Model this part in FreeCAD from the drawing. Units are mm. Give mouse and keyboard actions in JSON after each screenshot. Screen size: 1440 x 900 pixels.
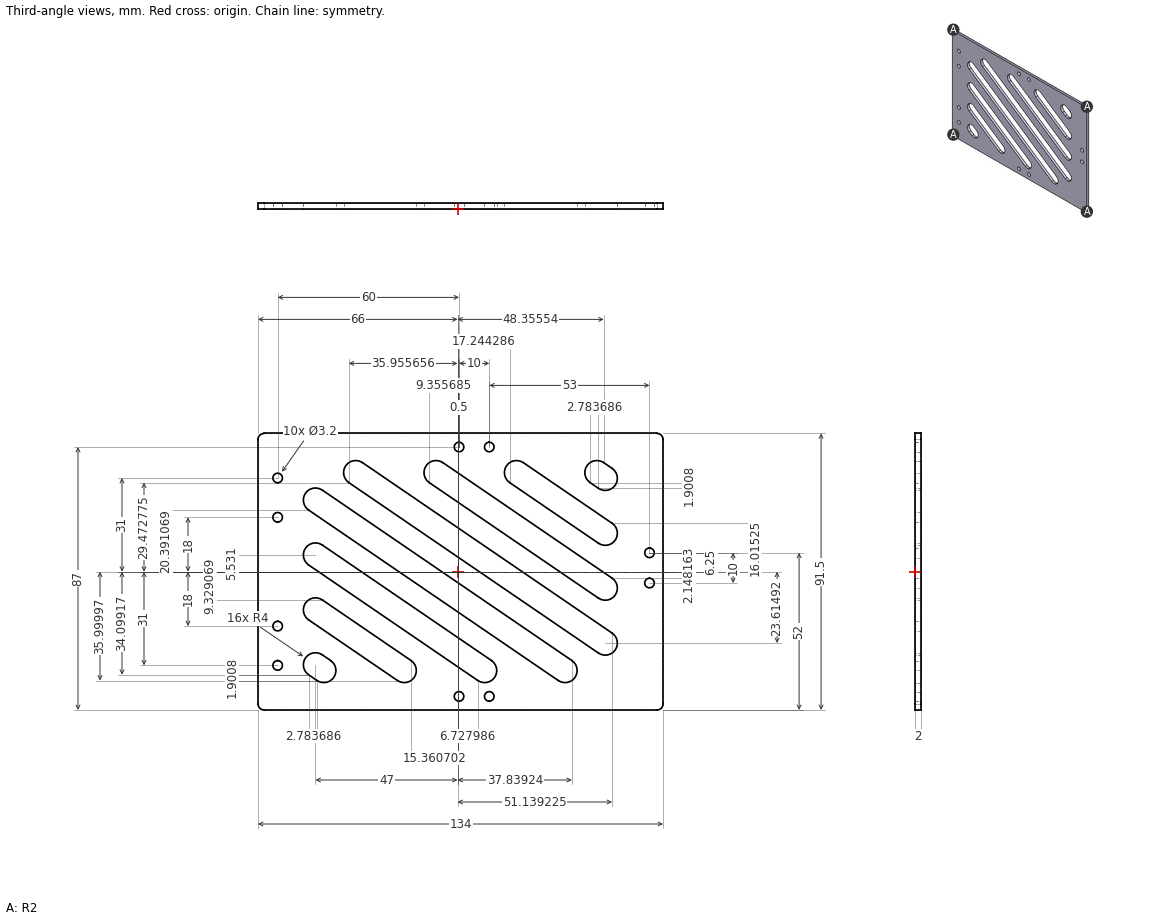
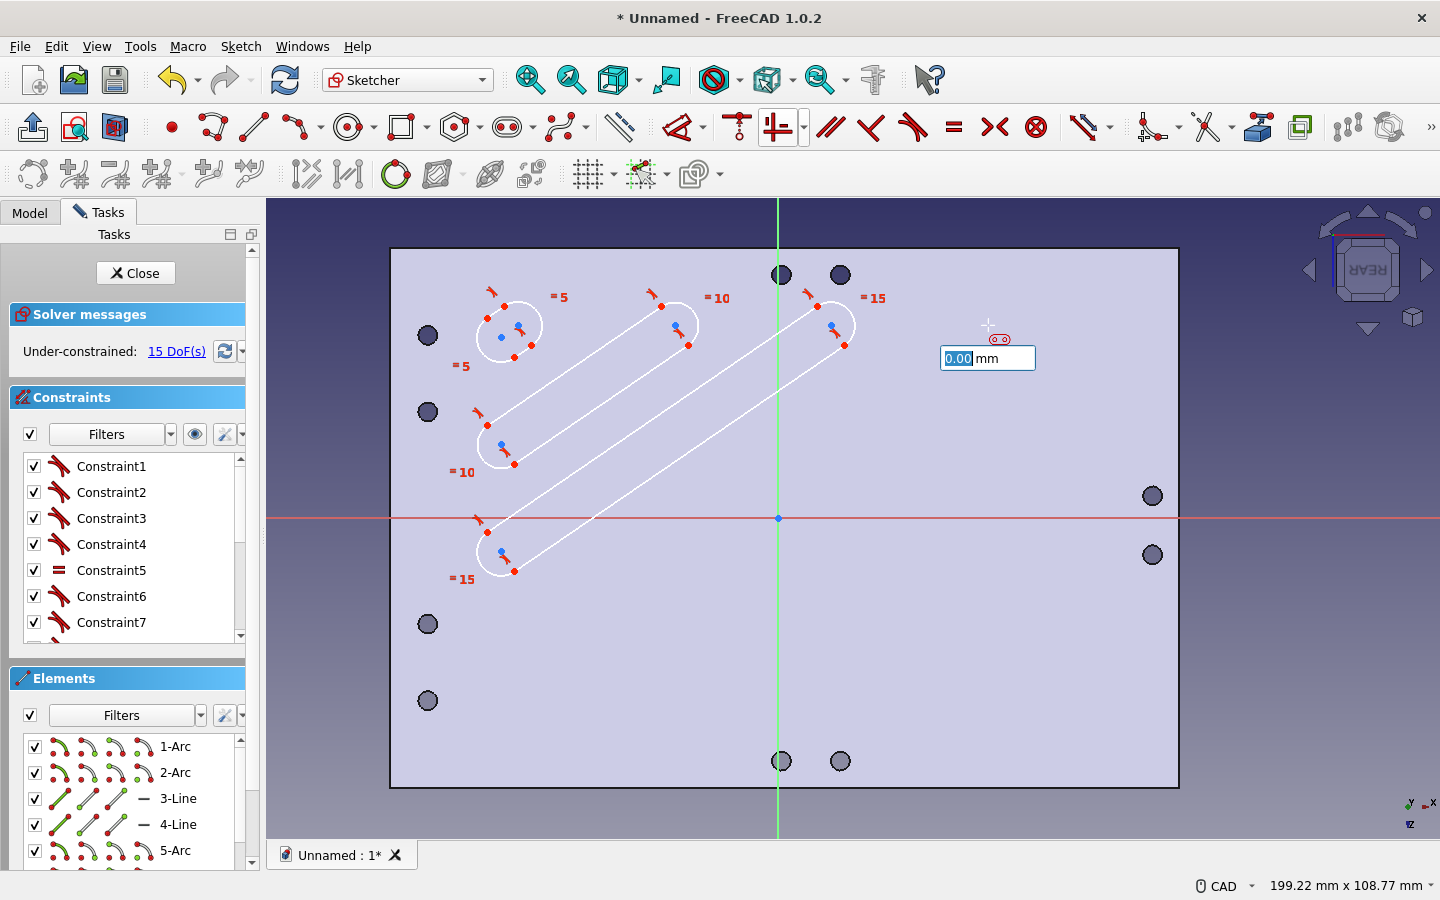
{"action": "left_click", "coordinate": [732, 472]}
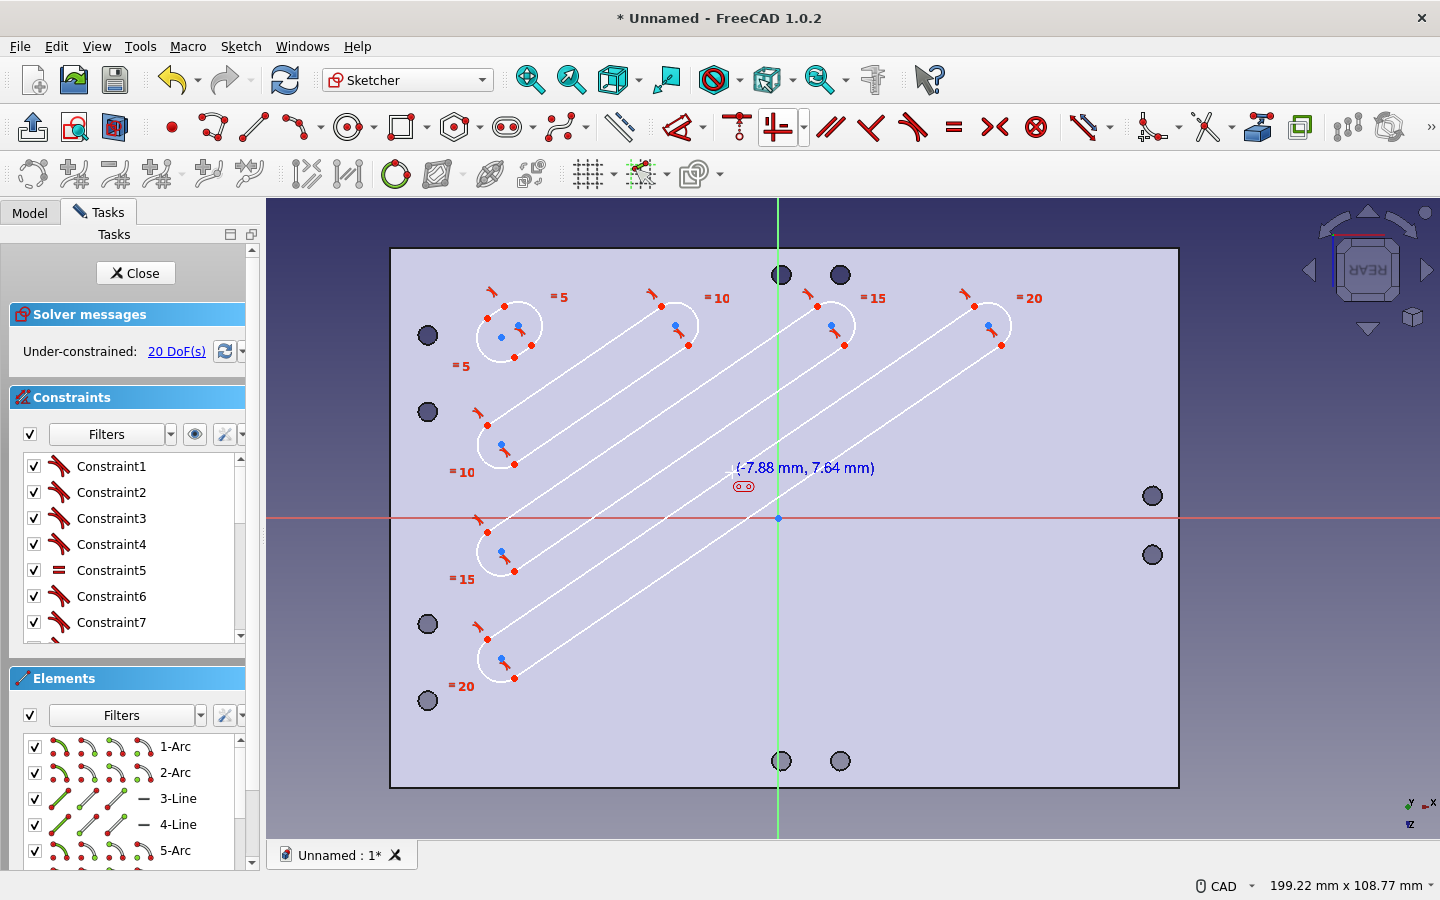
{"action": "left_click", "coordinate": [580, 711]}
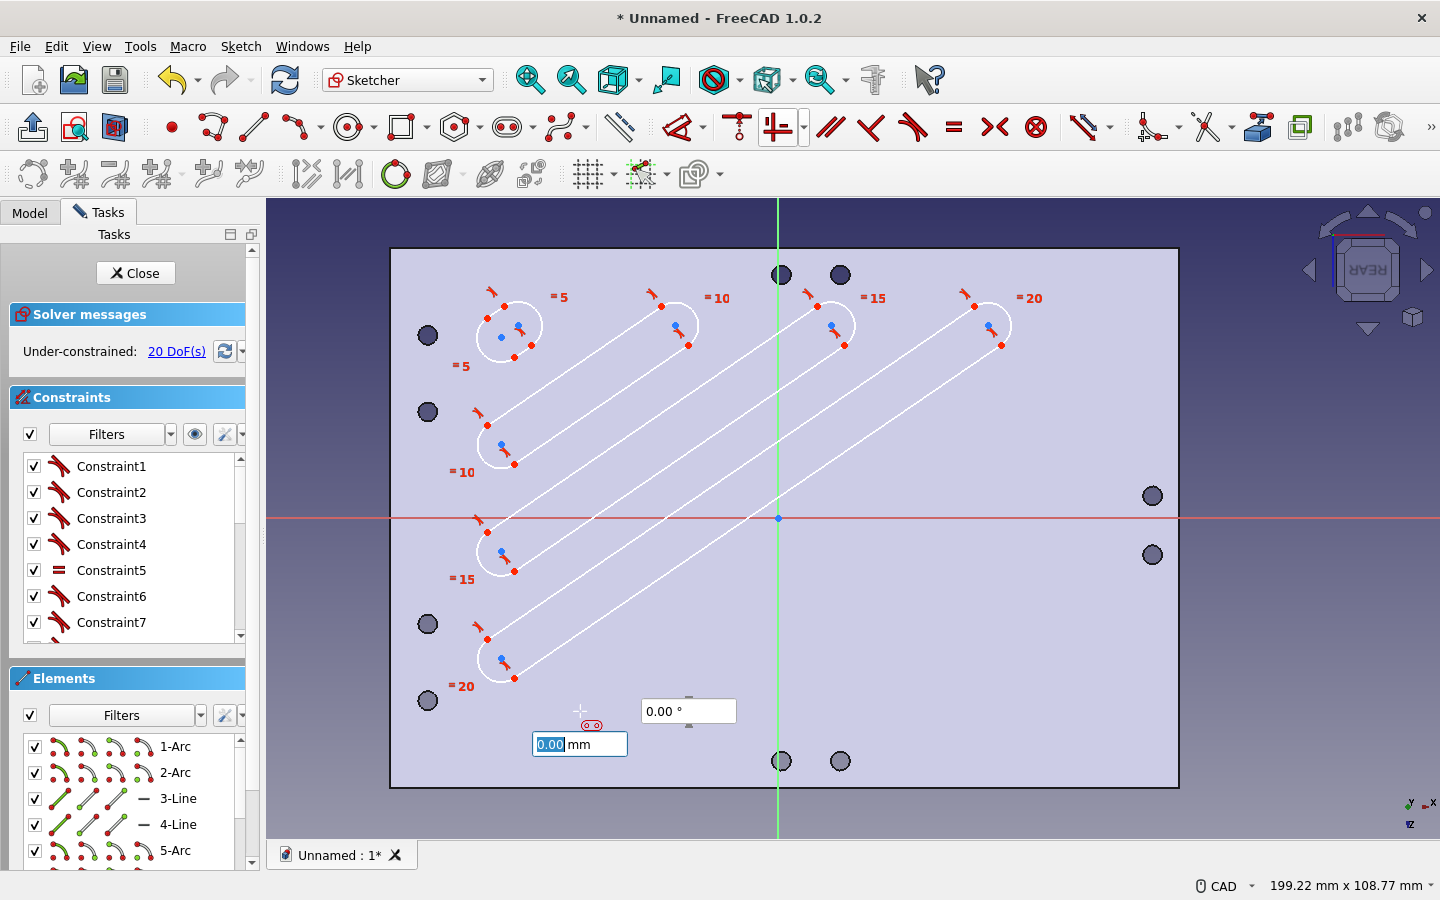
{"action": "left_click", "coordinate": [1067, 379]}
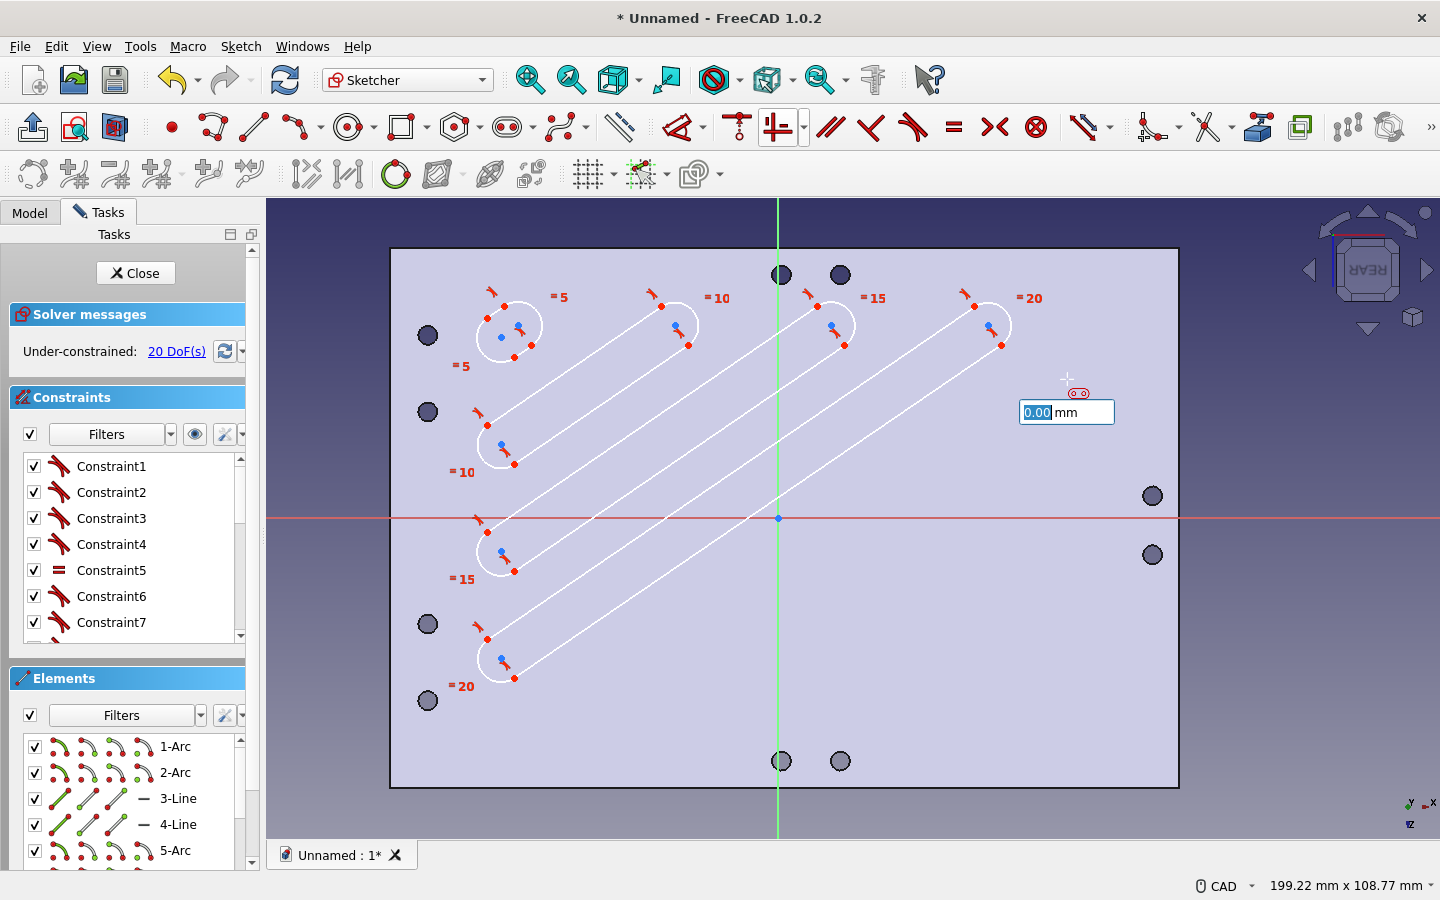
{"action": "left_click", "coordinate": [883, 476]}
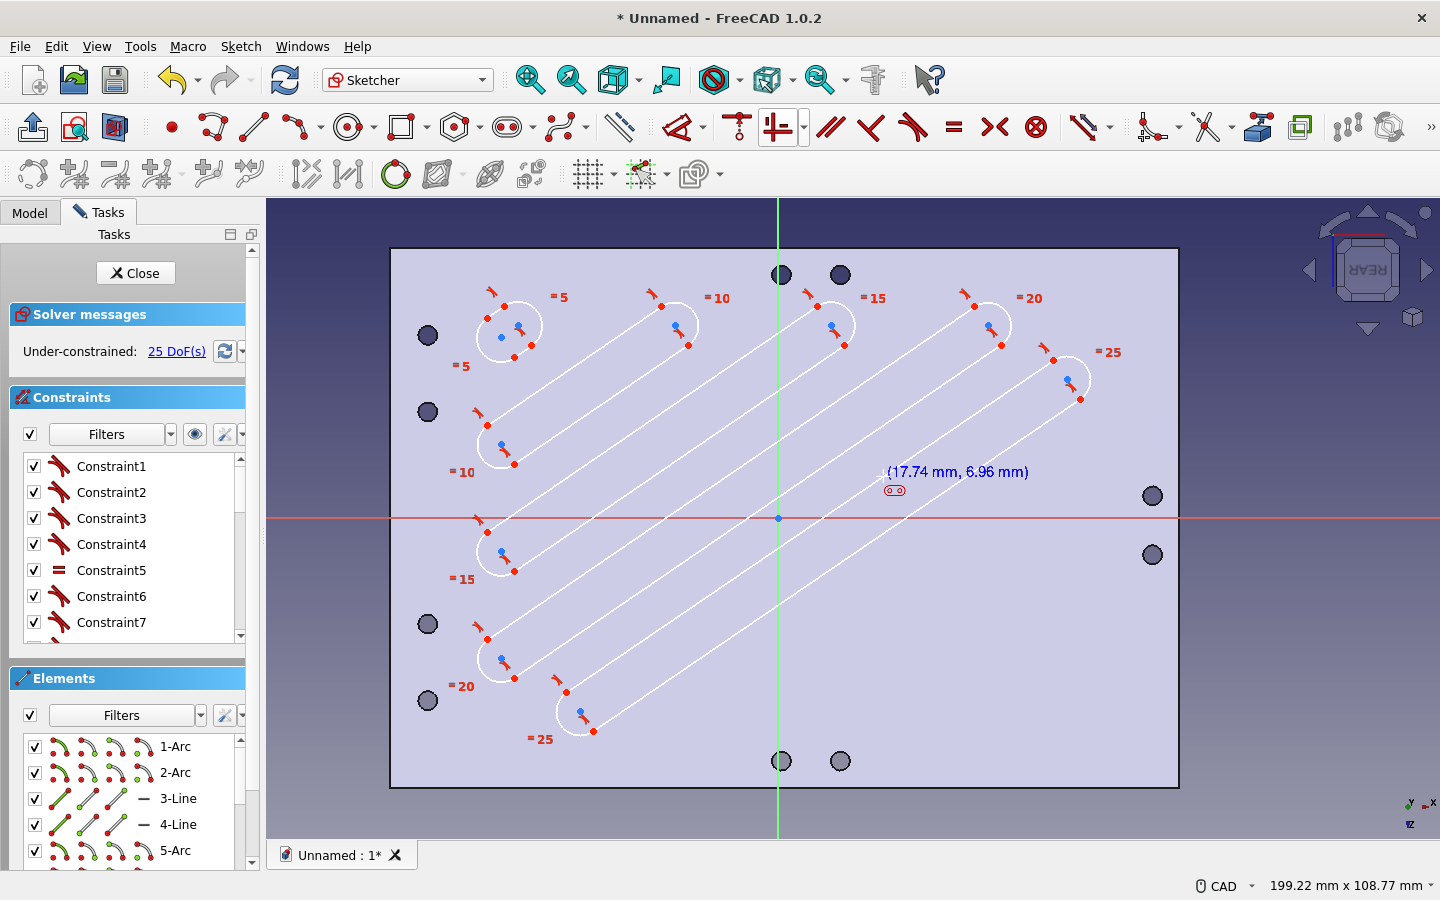
{"action": "left_click", "coordinate": [737, 711]}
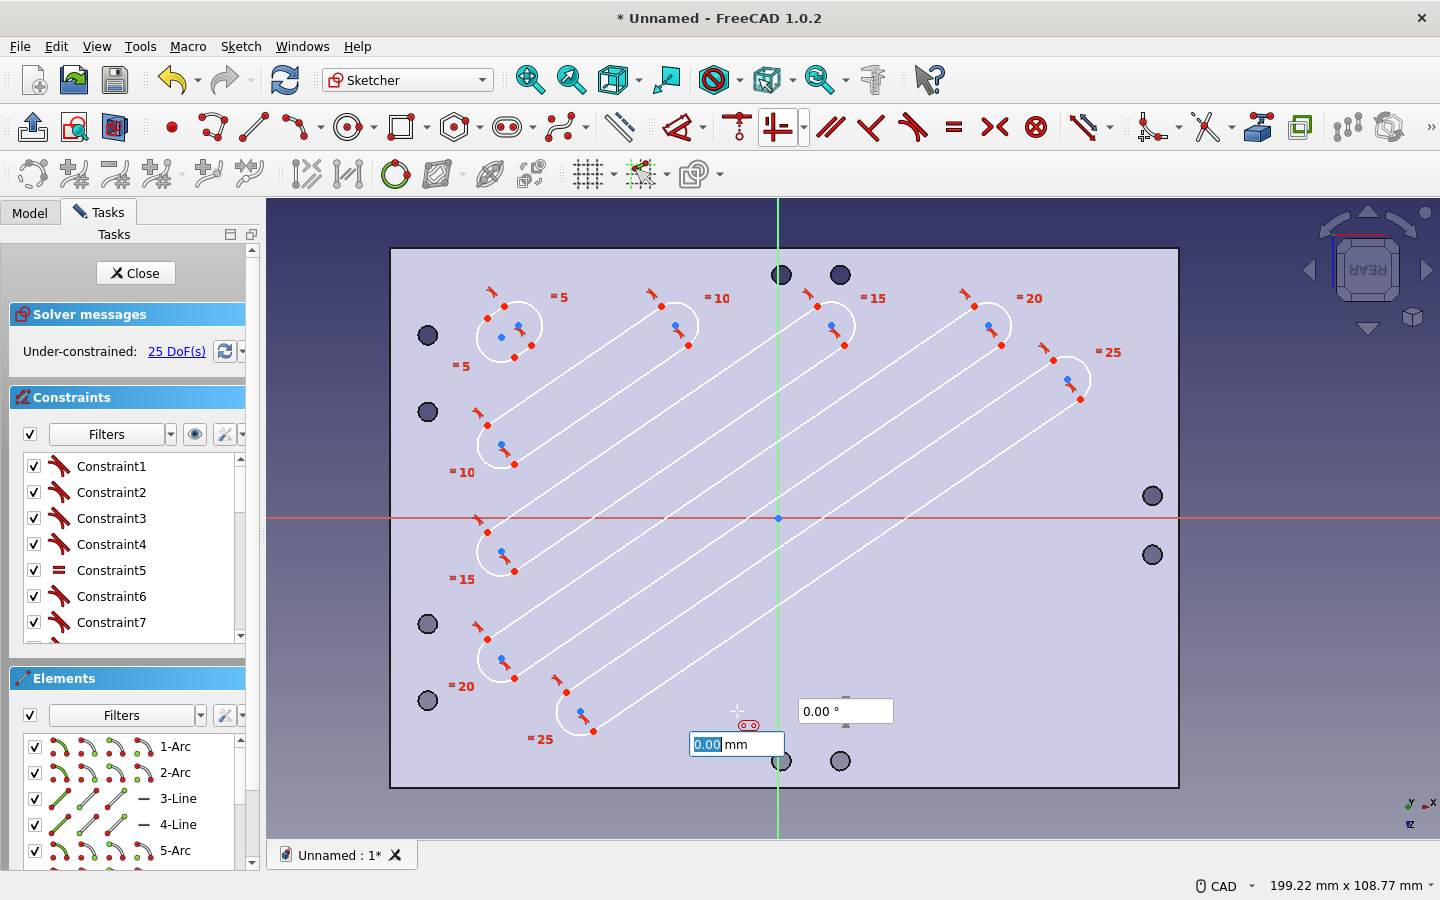
{"action": "left_click", "coordinate": [1067, 486]}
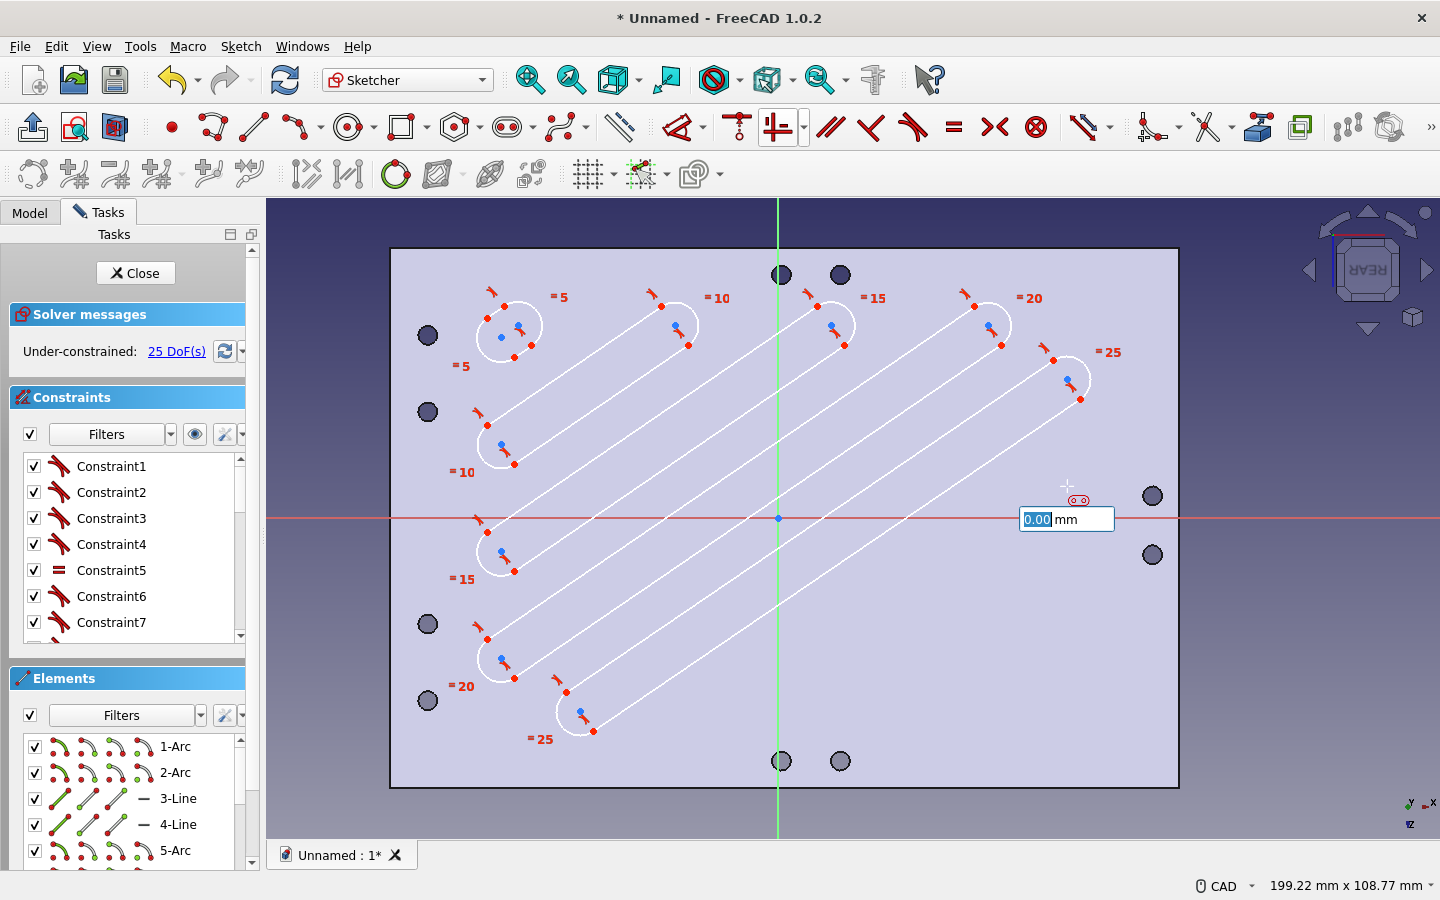
{"action": "left_click", "coordinate": [888, 579]}